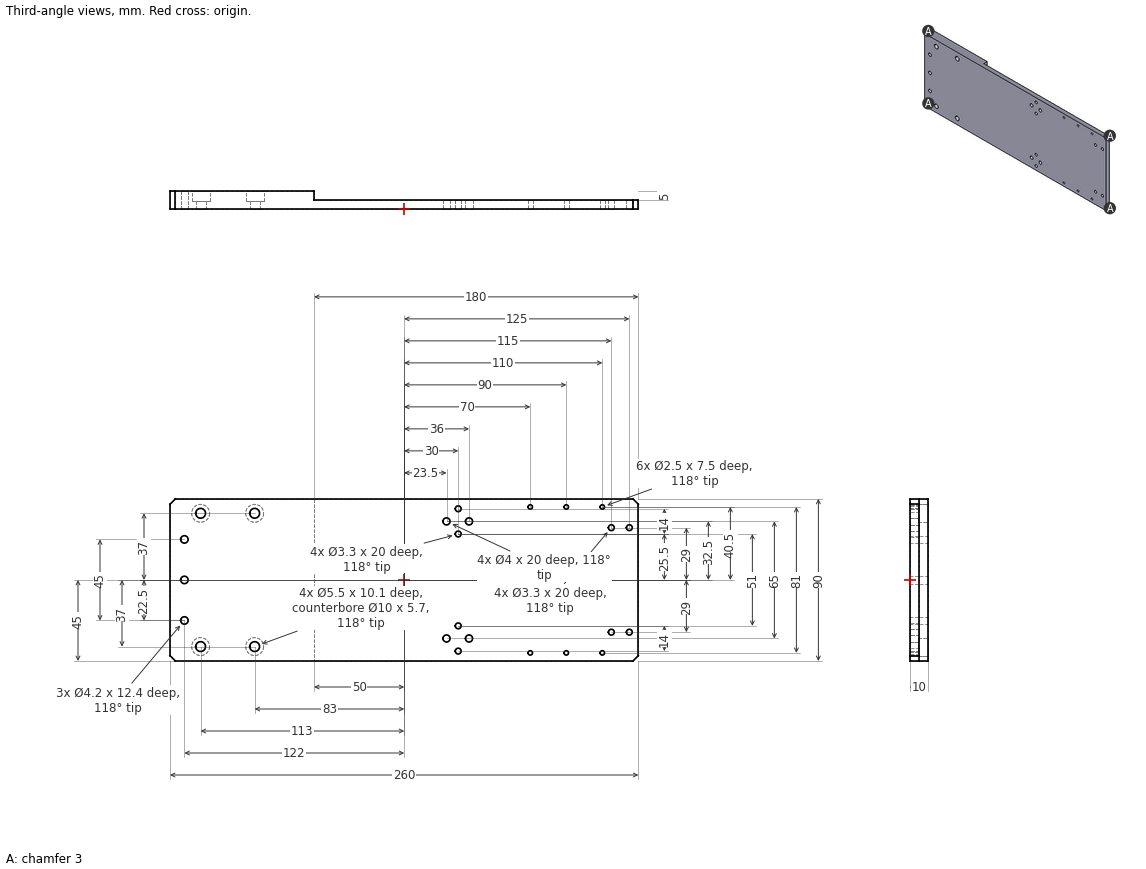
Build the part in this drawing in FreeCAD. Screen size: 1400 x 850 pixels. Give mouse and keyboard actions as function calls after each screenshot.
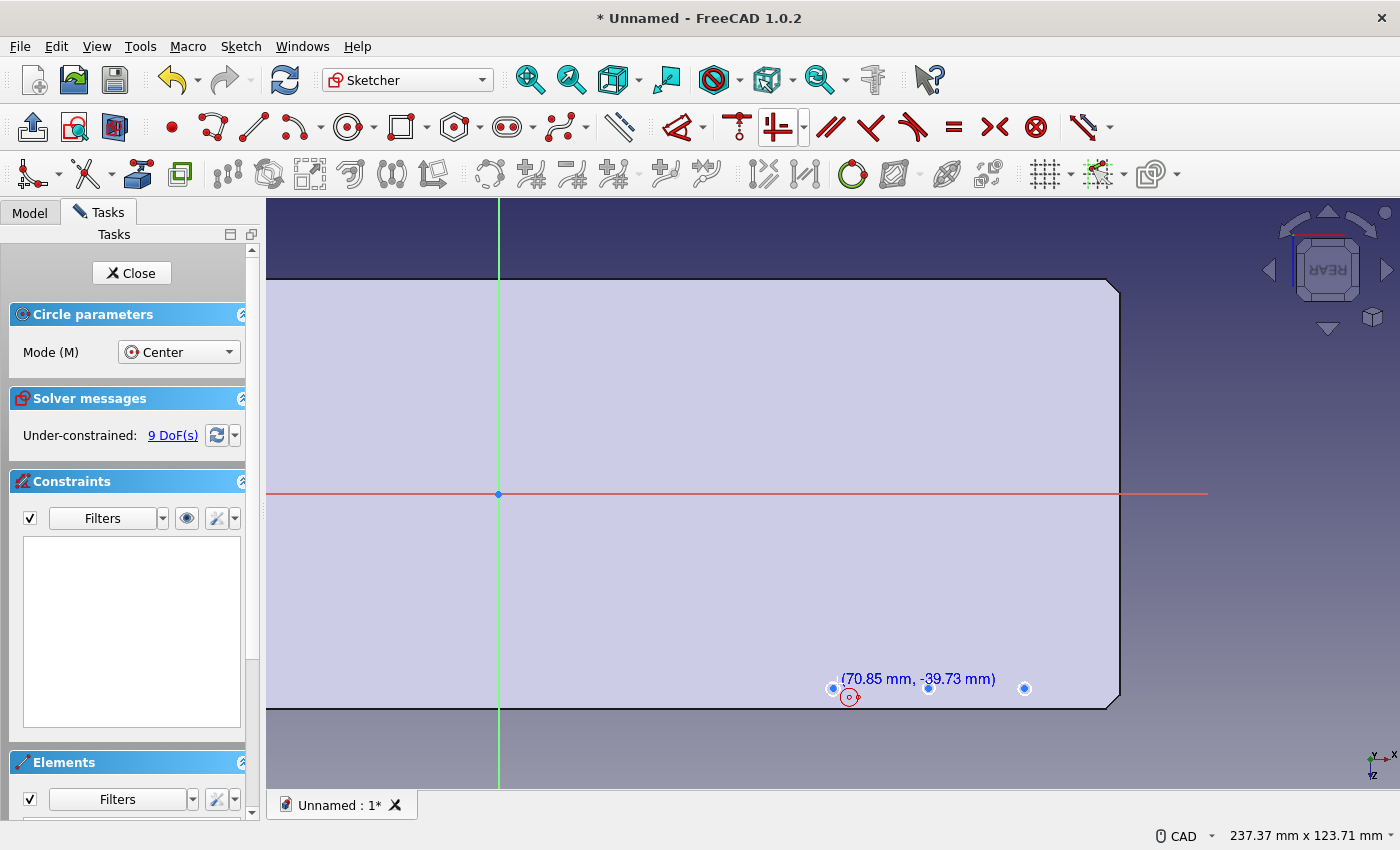
scroll(1024, 301, up, 7)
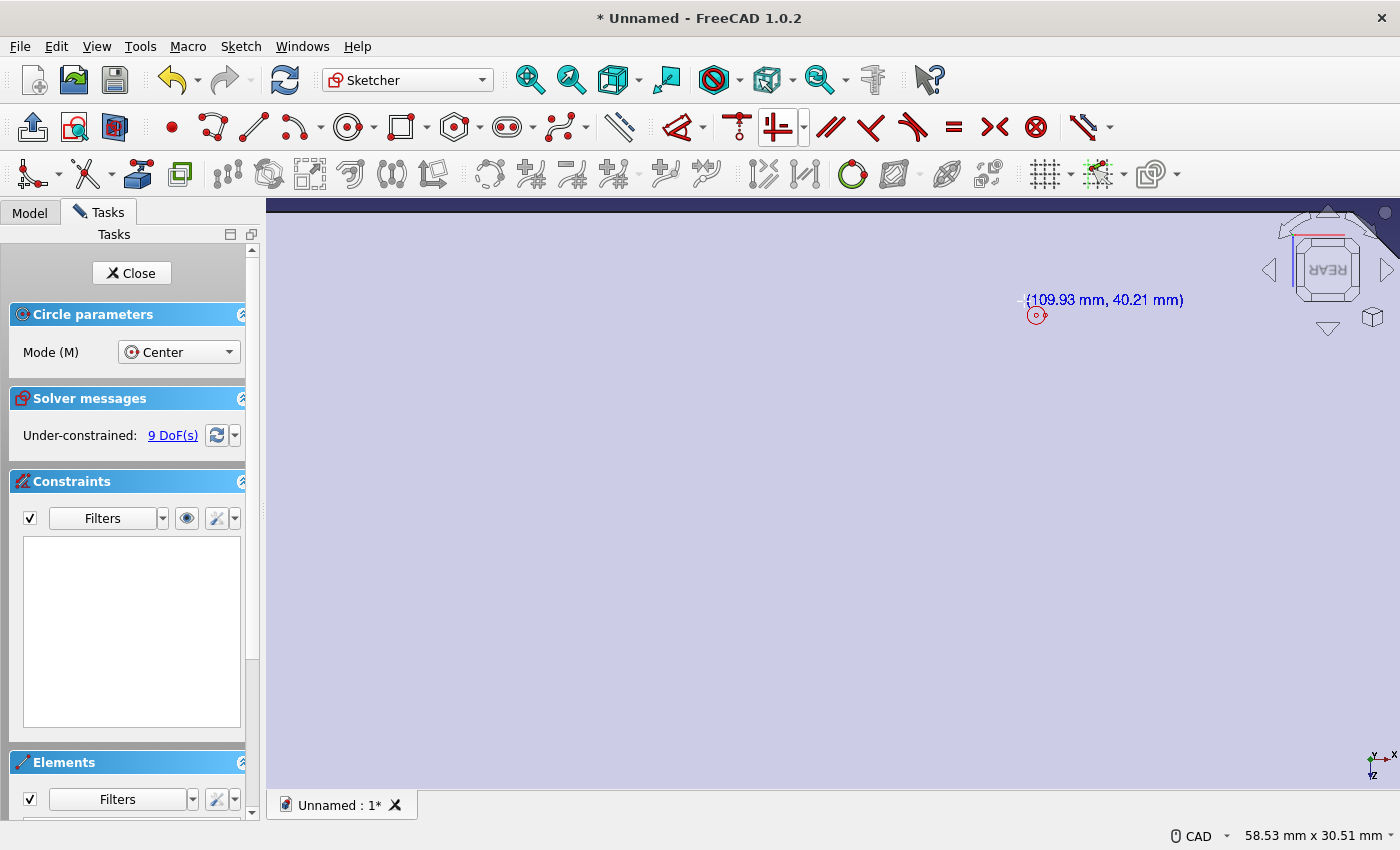
scroll(1025, 300, down, 7)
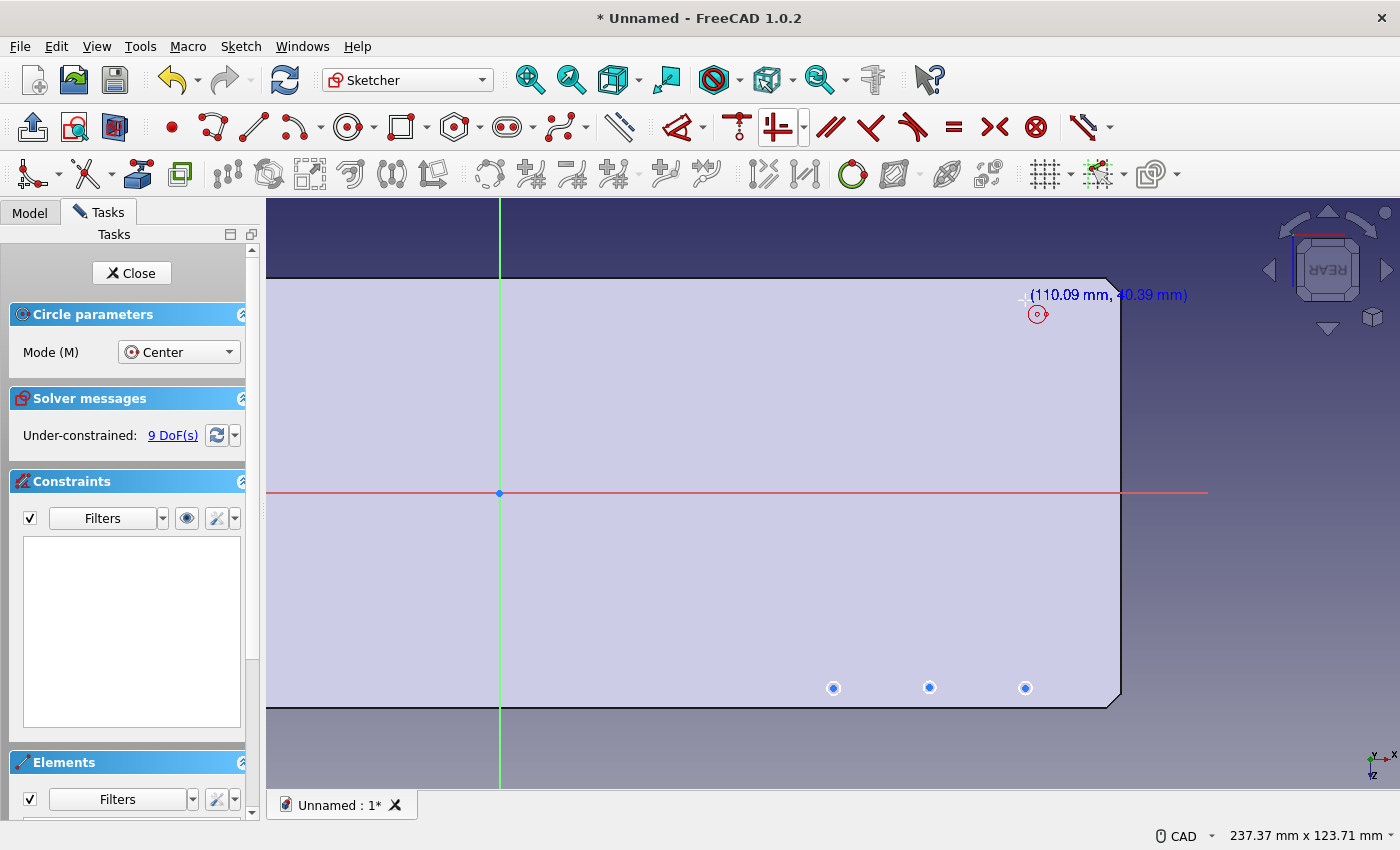
click(1025, 300)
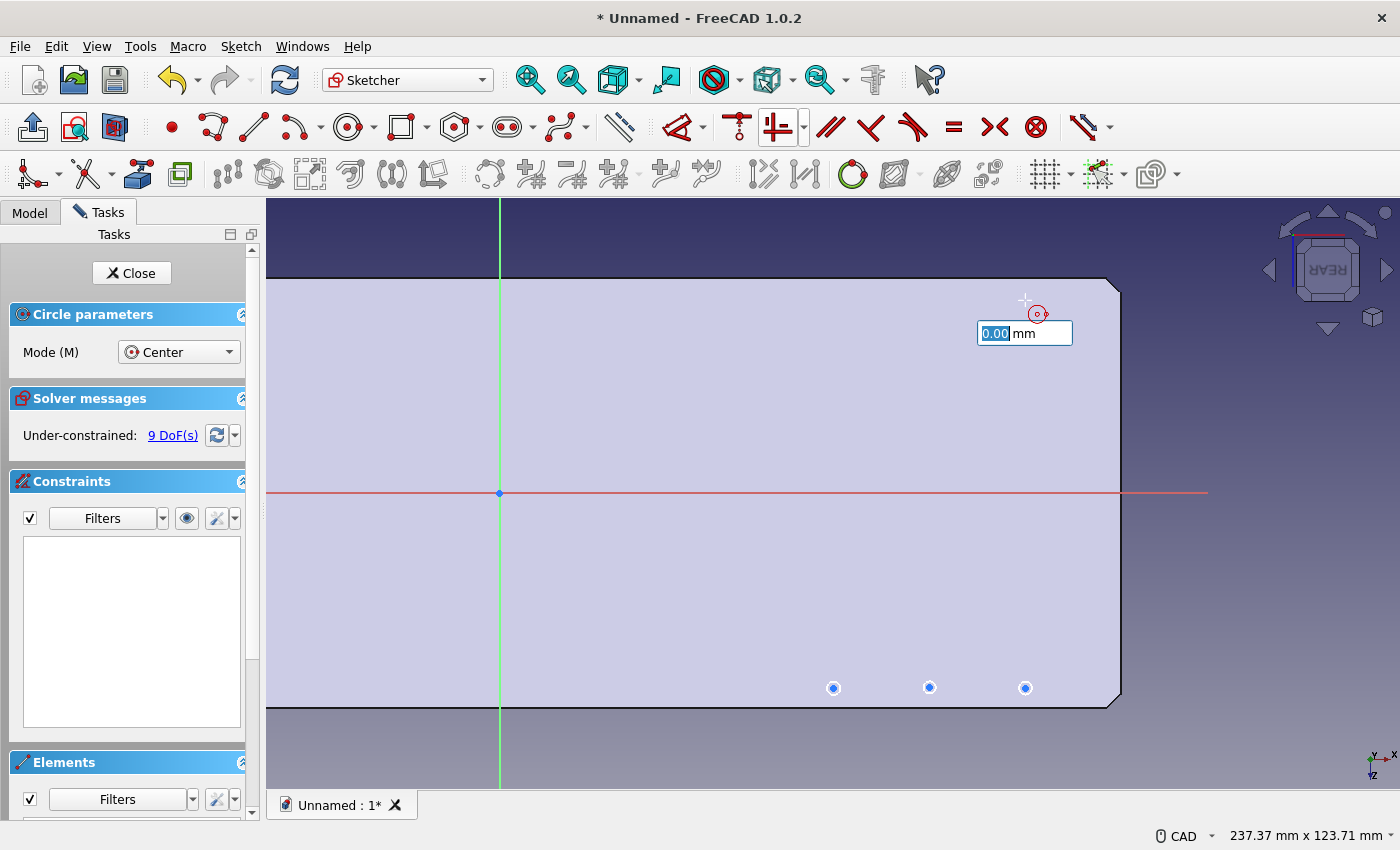
scroll(1029, 296, up, 5)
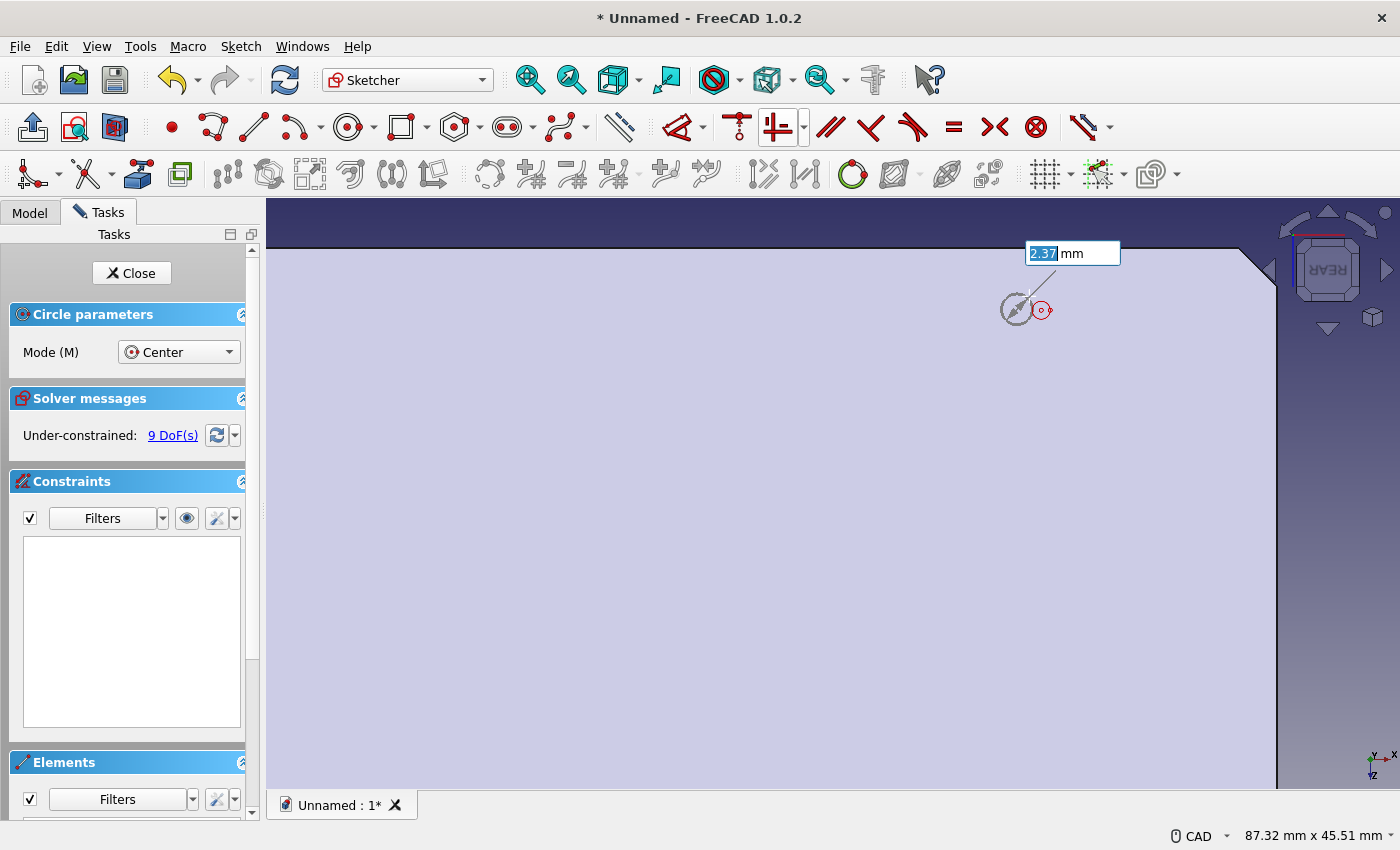
click(1029, 295)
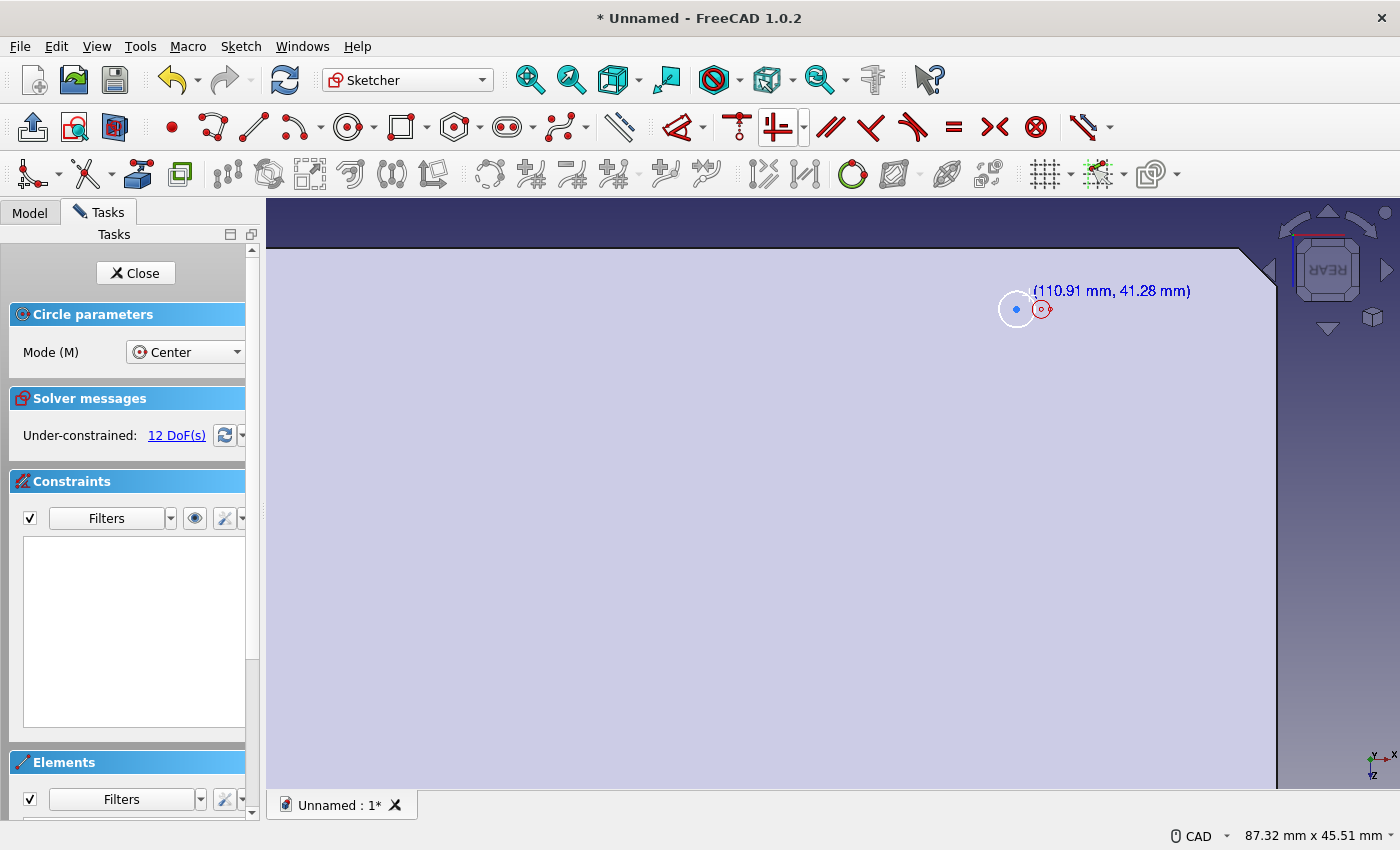
scroll(757, 306, up, 2)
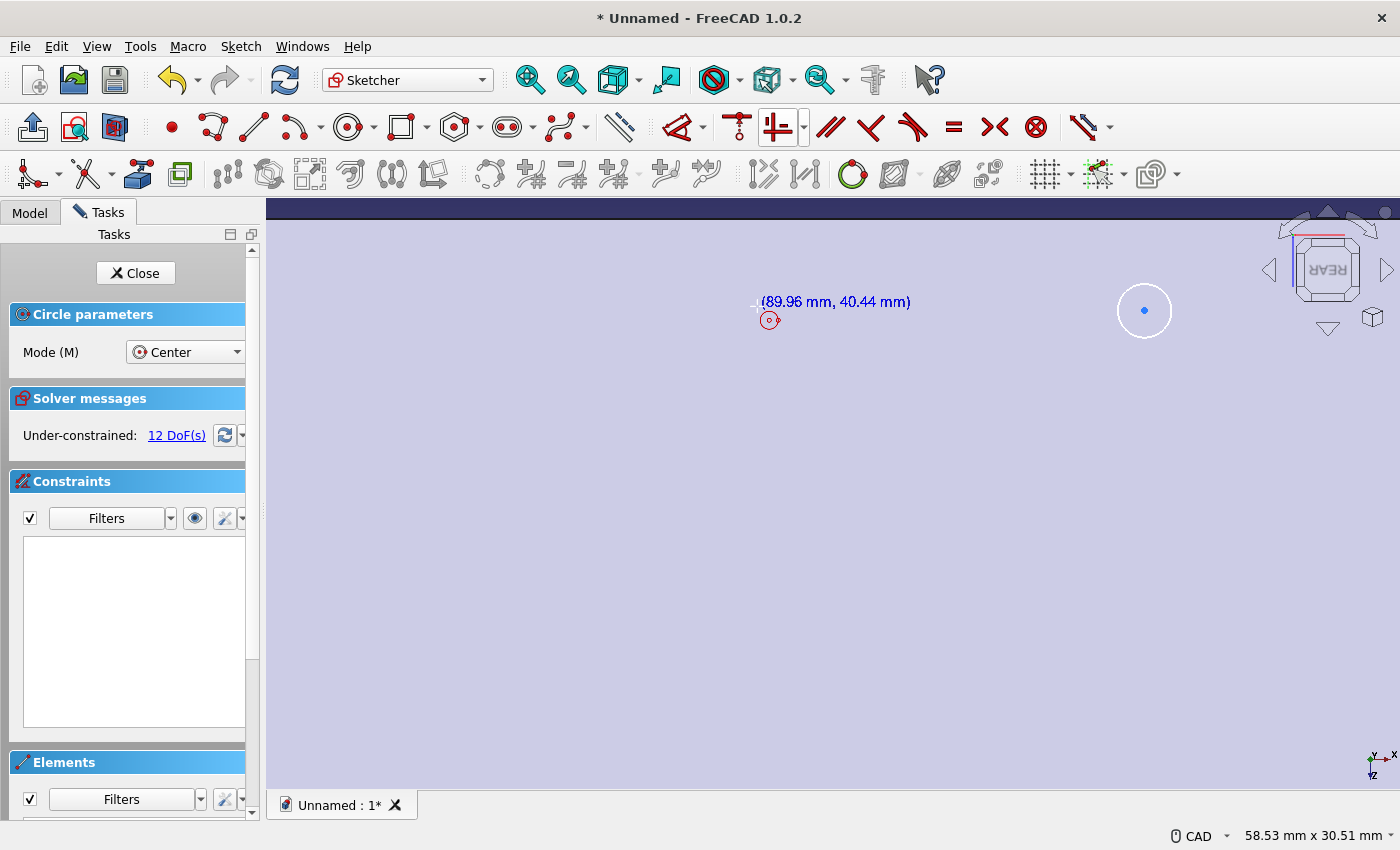
scroll(985, 298, down, 7)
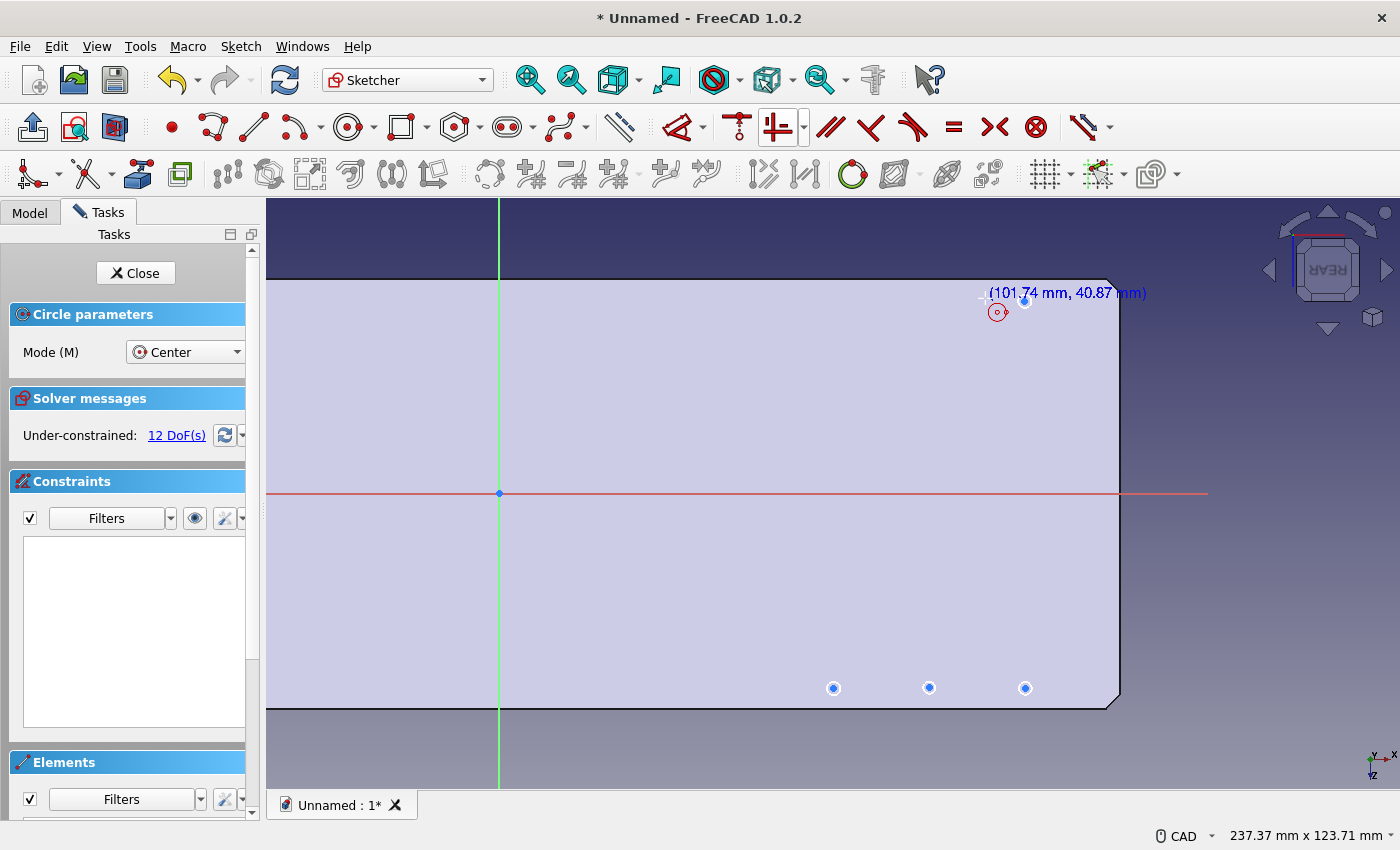
click(929, 300)